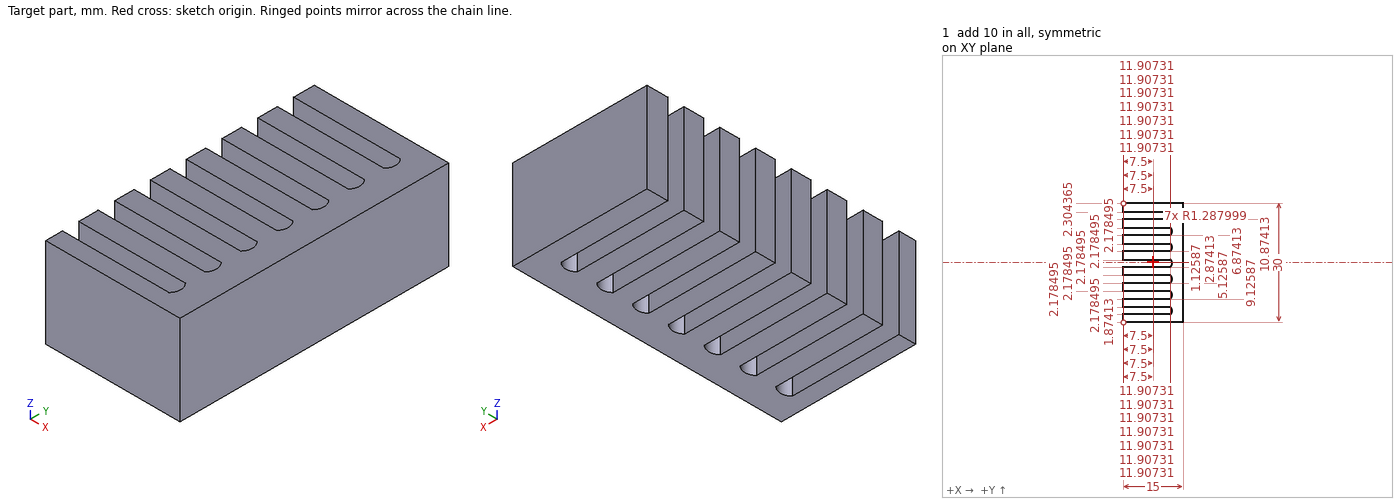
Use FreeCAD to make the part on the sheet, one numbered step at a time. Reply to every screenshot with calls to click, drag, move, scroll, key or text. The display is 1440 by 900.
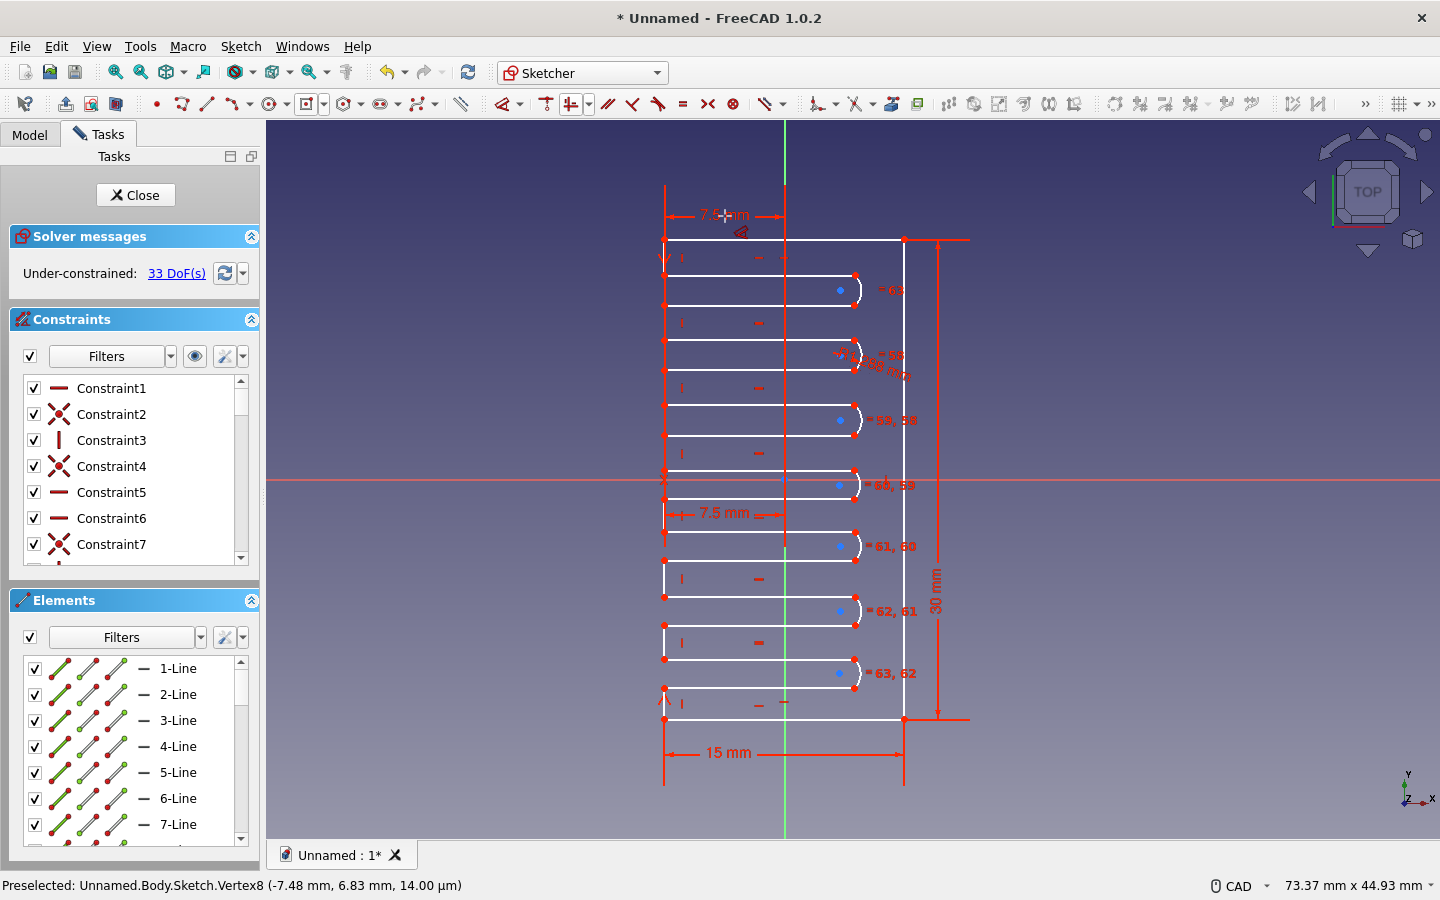
click(665, 436)
click(725, 354)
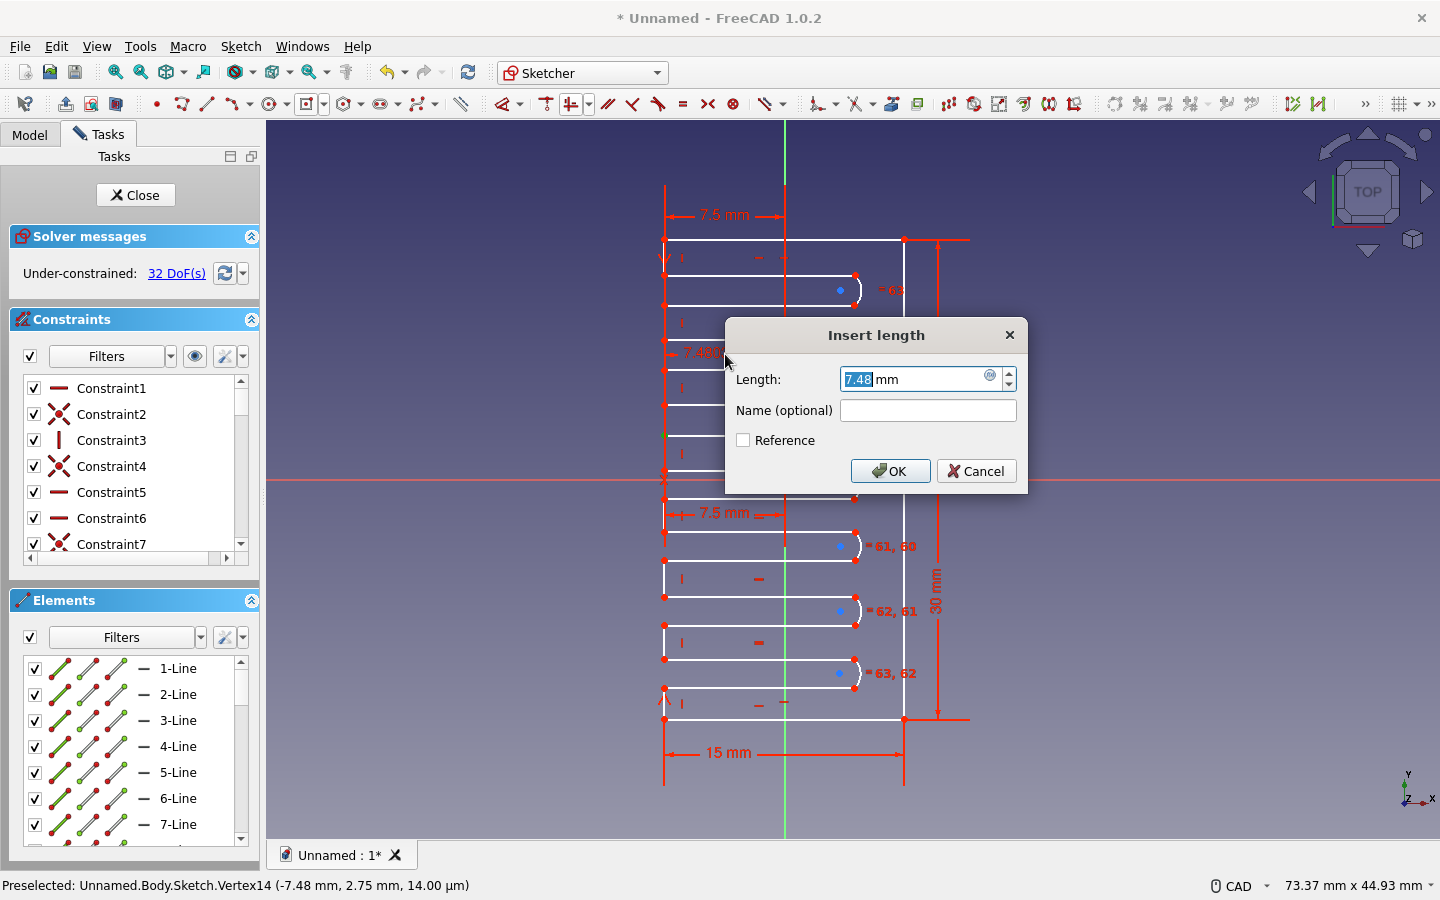
text(7.5)
key(Return)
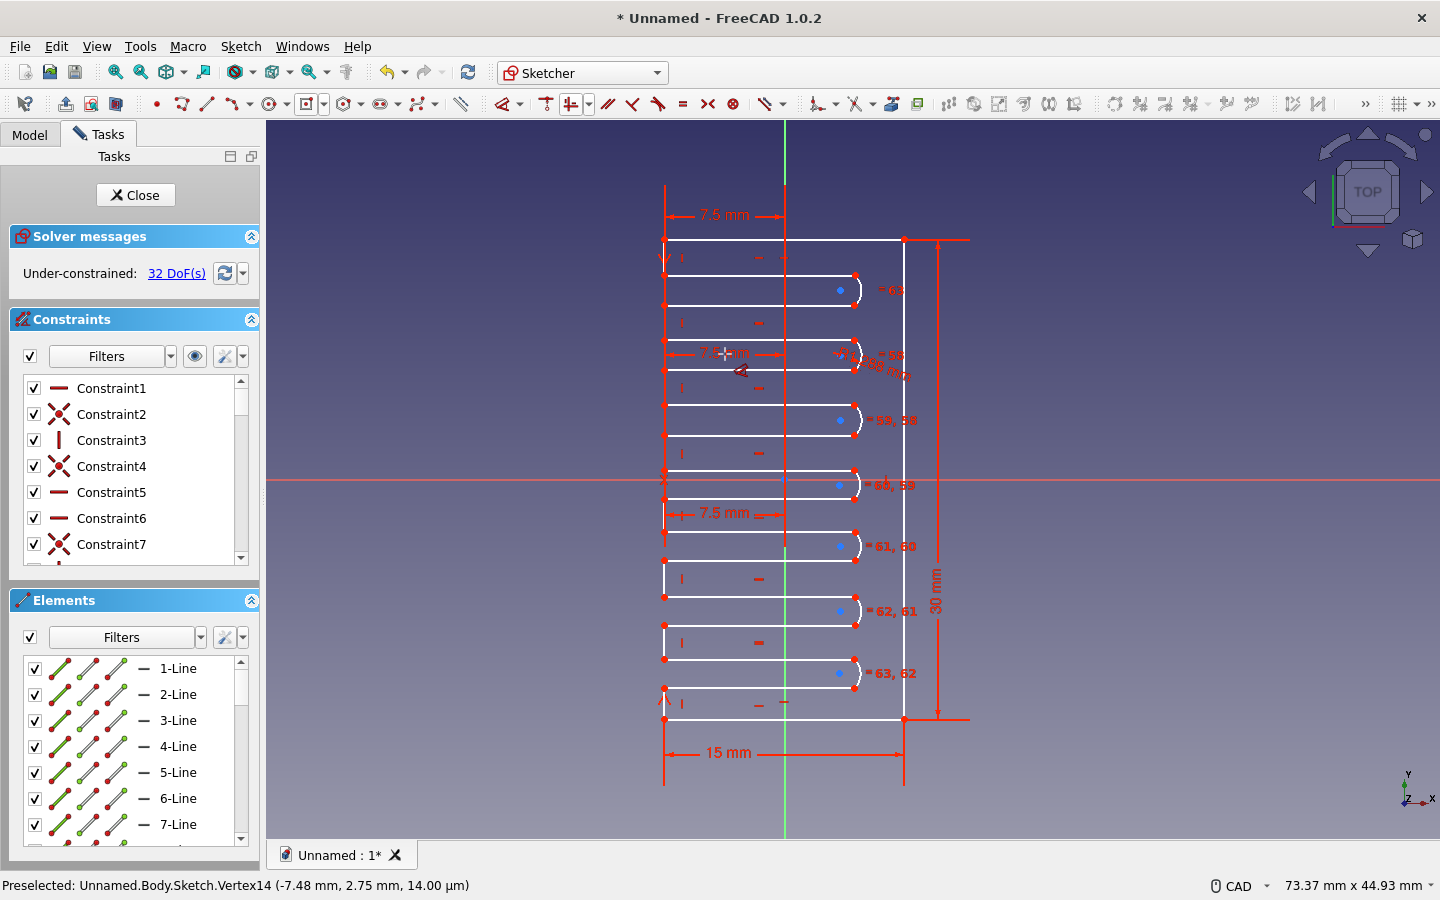
click(664, 499)
click(725, 422)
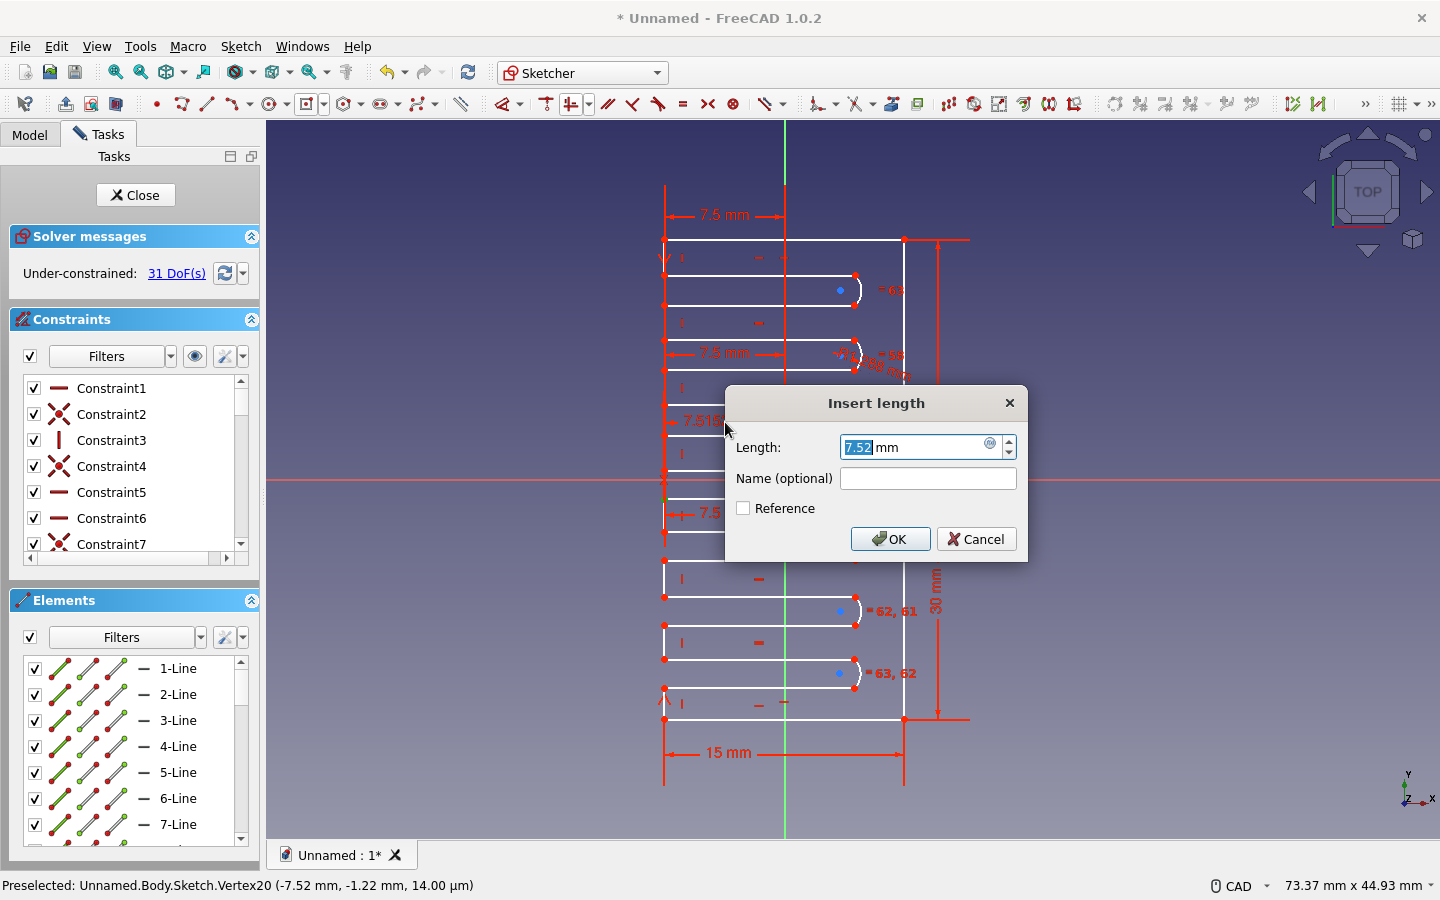
text(7.5)
key(Return)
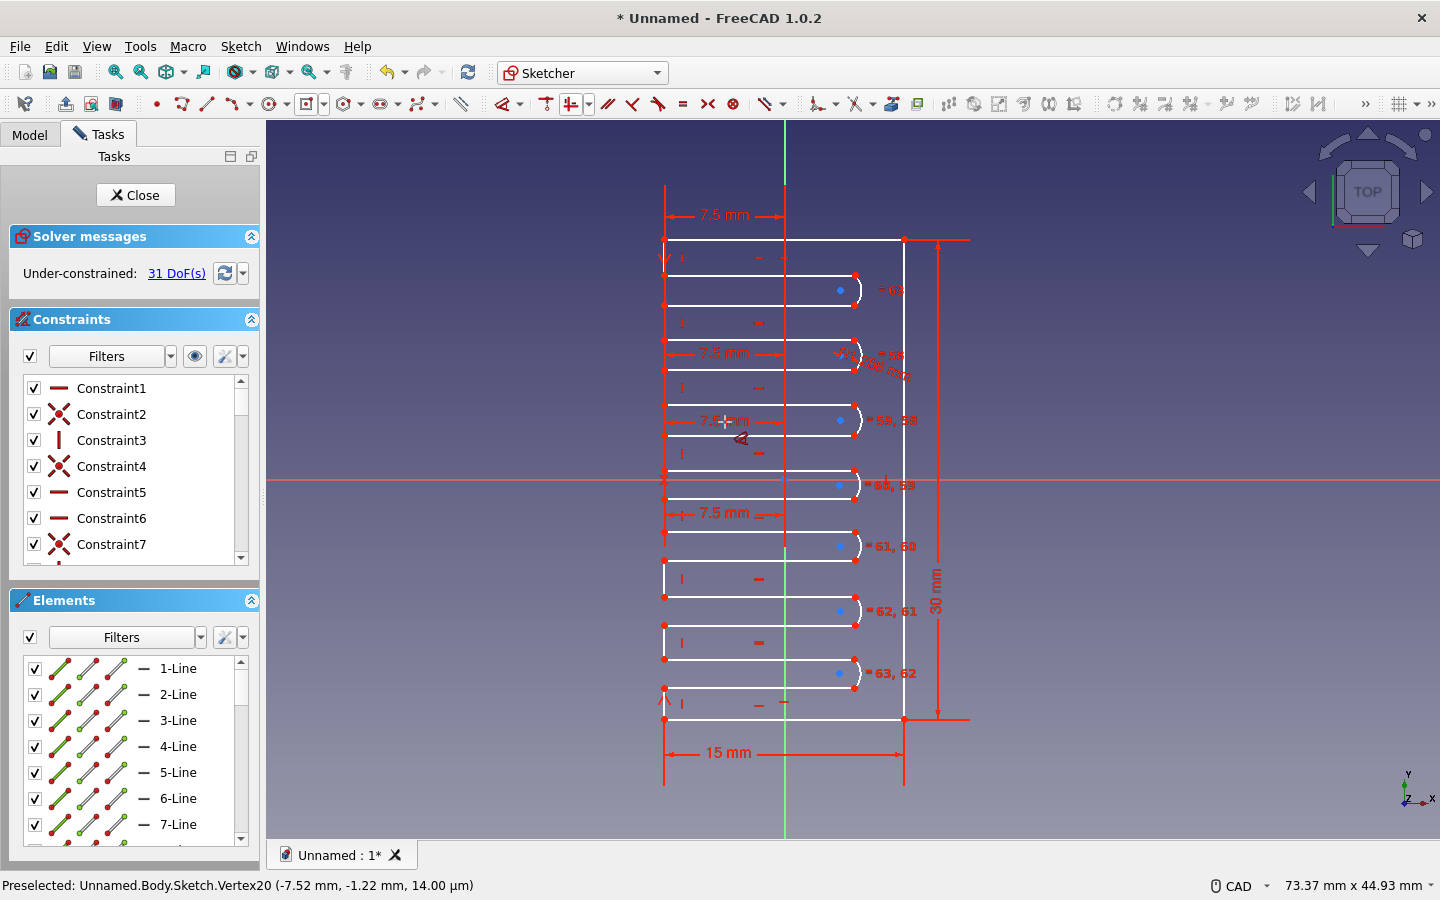
click(664, 561)
click(725, 643)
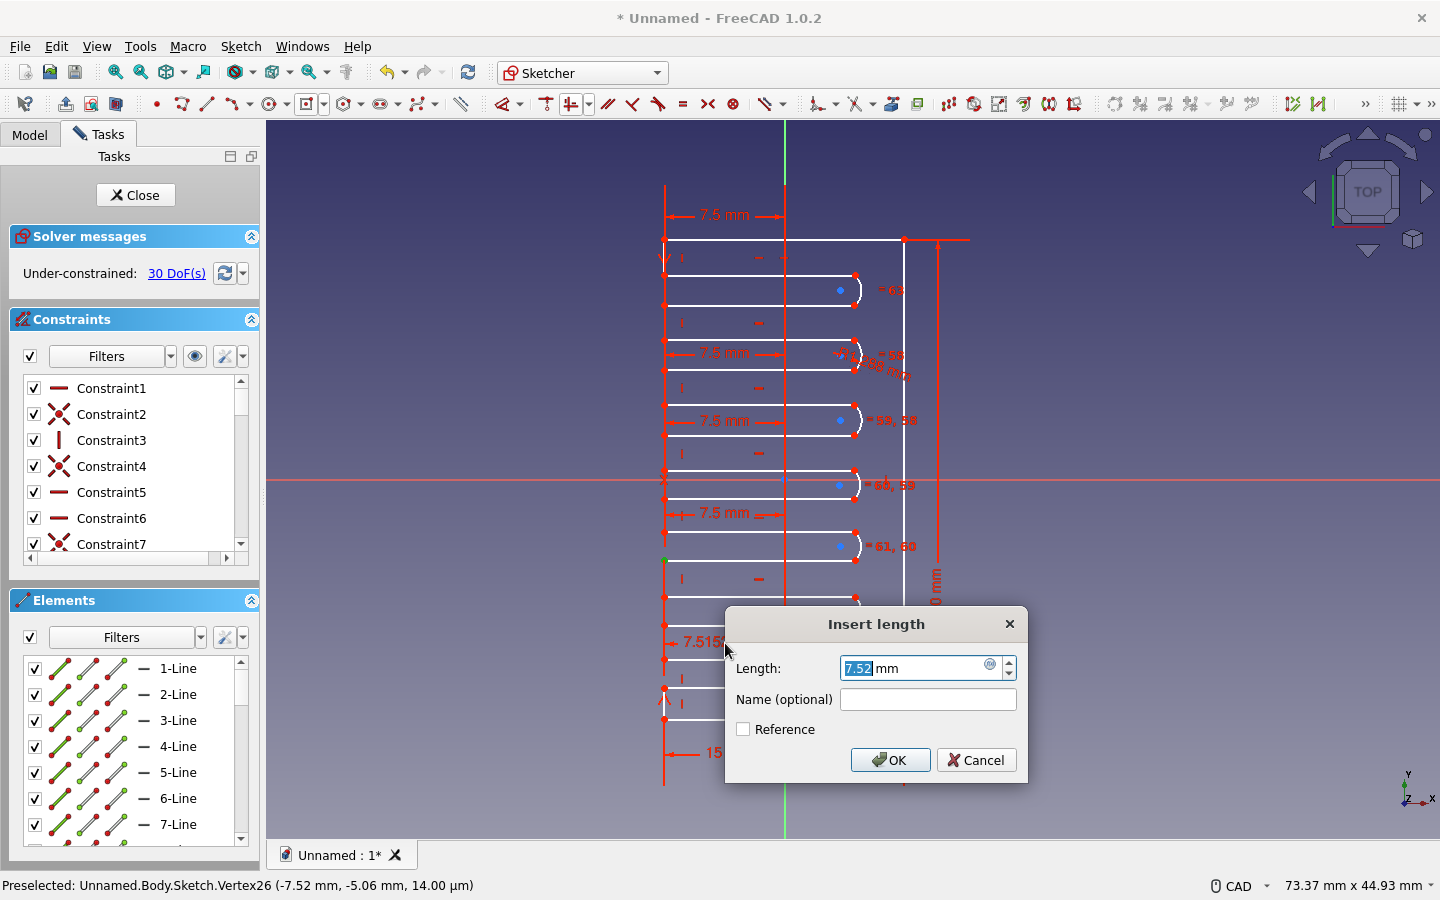
text(7.5)
key(Return)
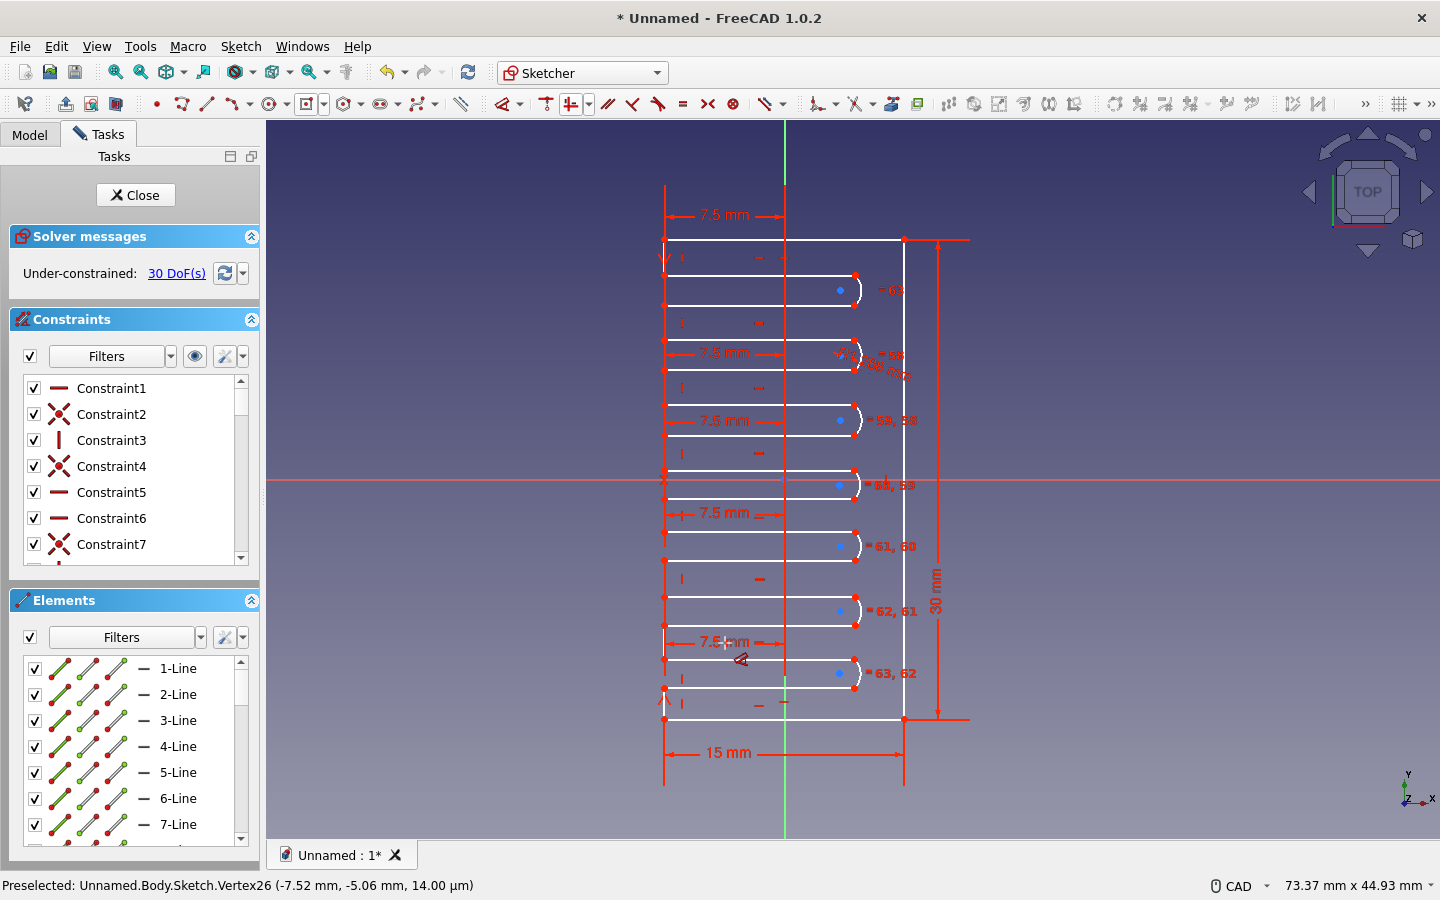
click(664, 626)
click(725, 780)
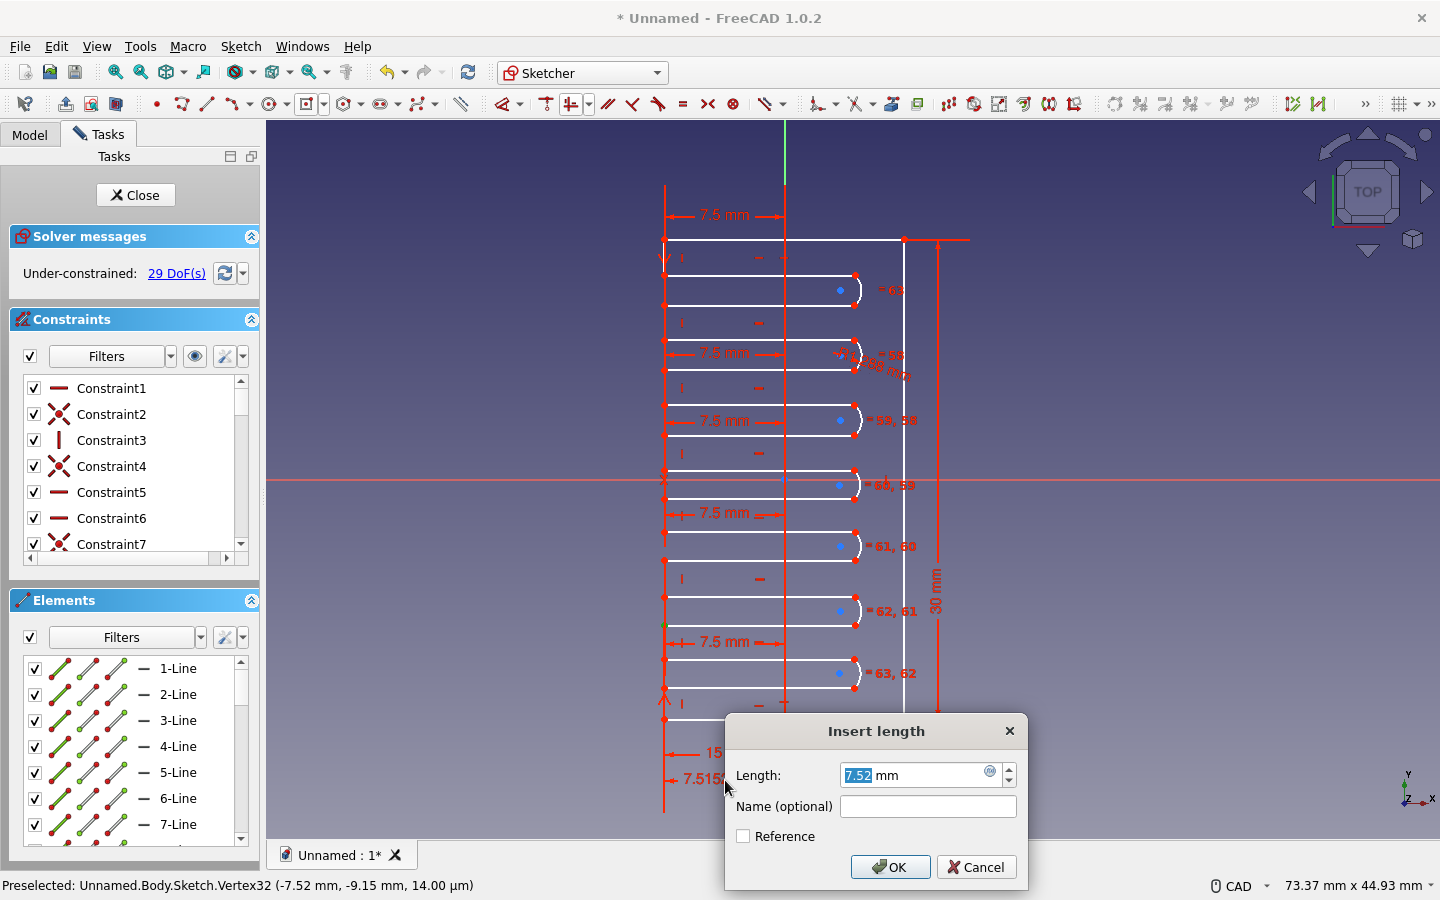
text(7.5)
key(Return)